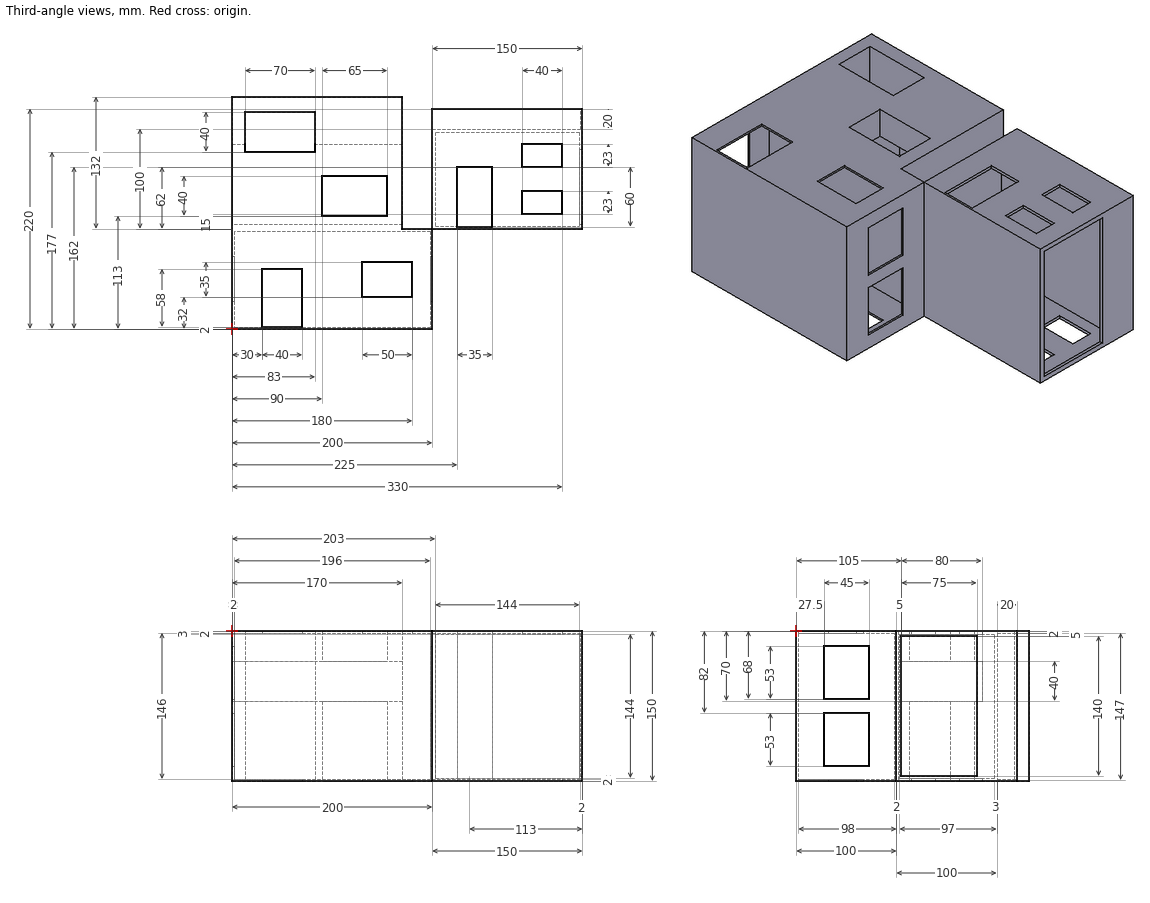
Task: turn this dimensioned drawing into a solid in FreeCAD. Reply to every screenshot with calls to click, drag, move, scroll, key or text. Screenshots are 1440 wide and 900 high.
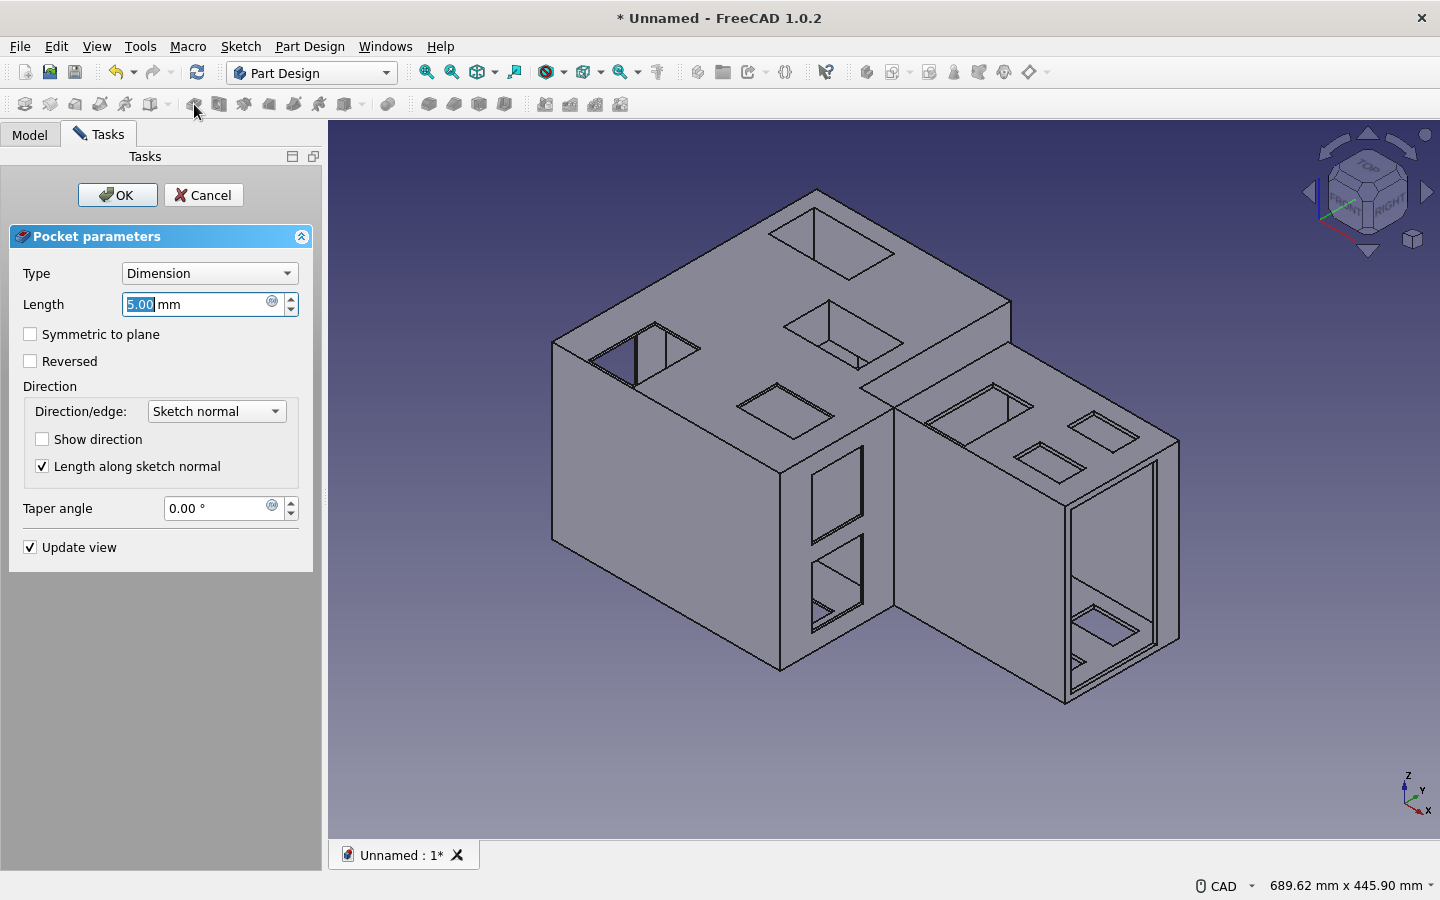
text(113)
key(Tab)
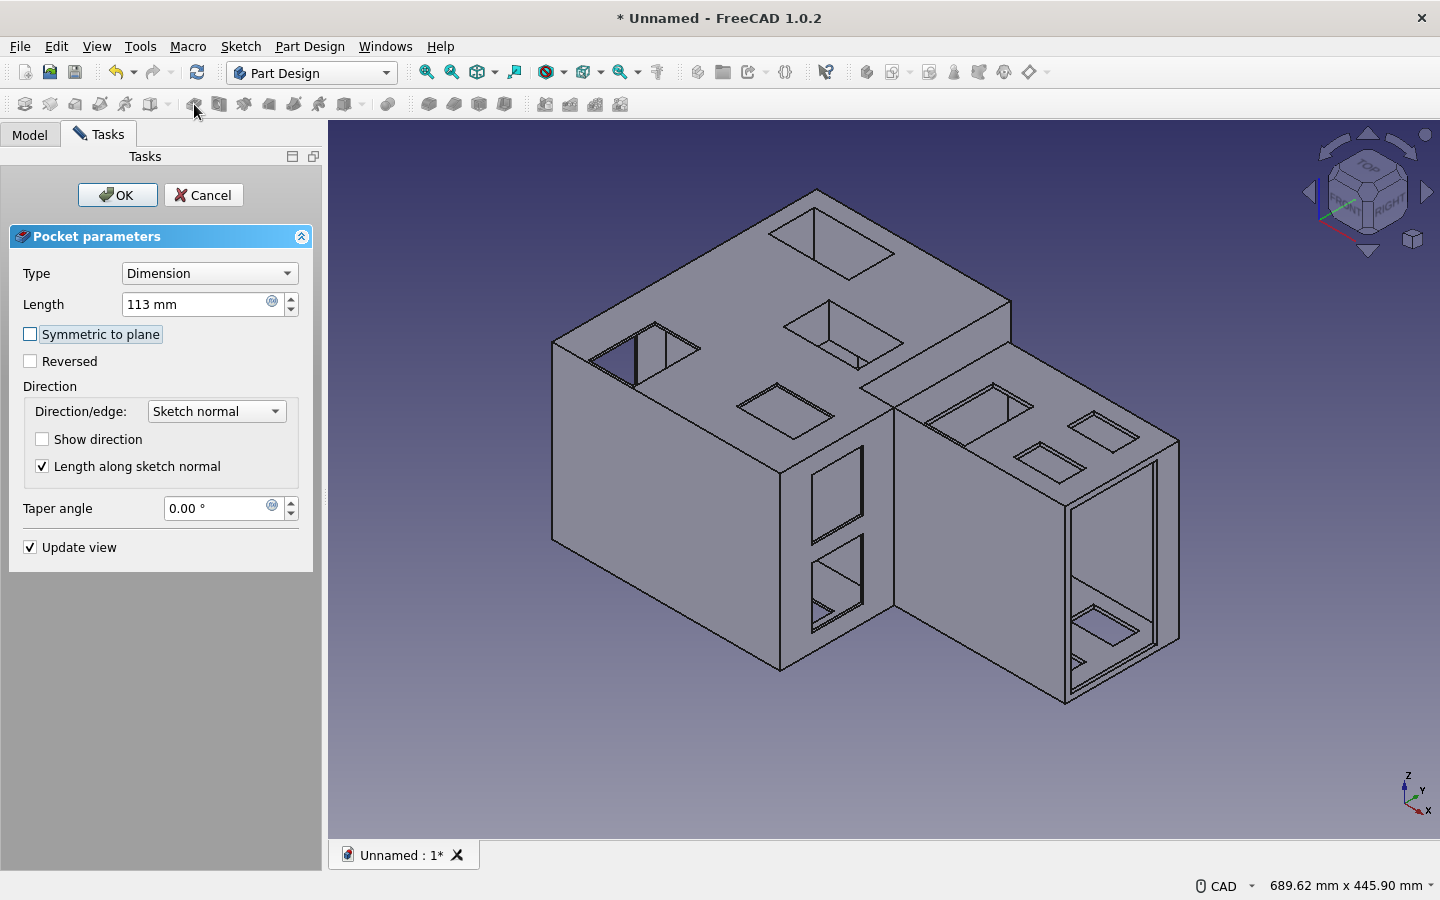
click(118, 195)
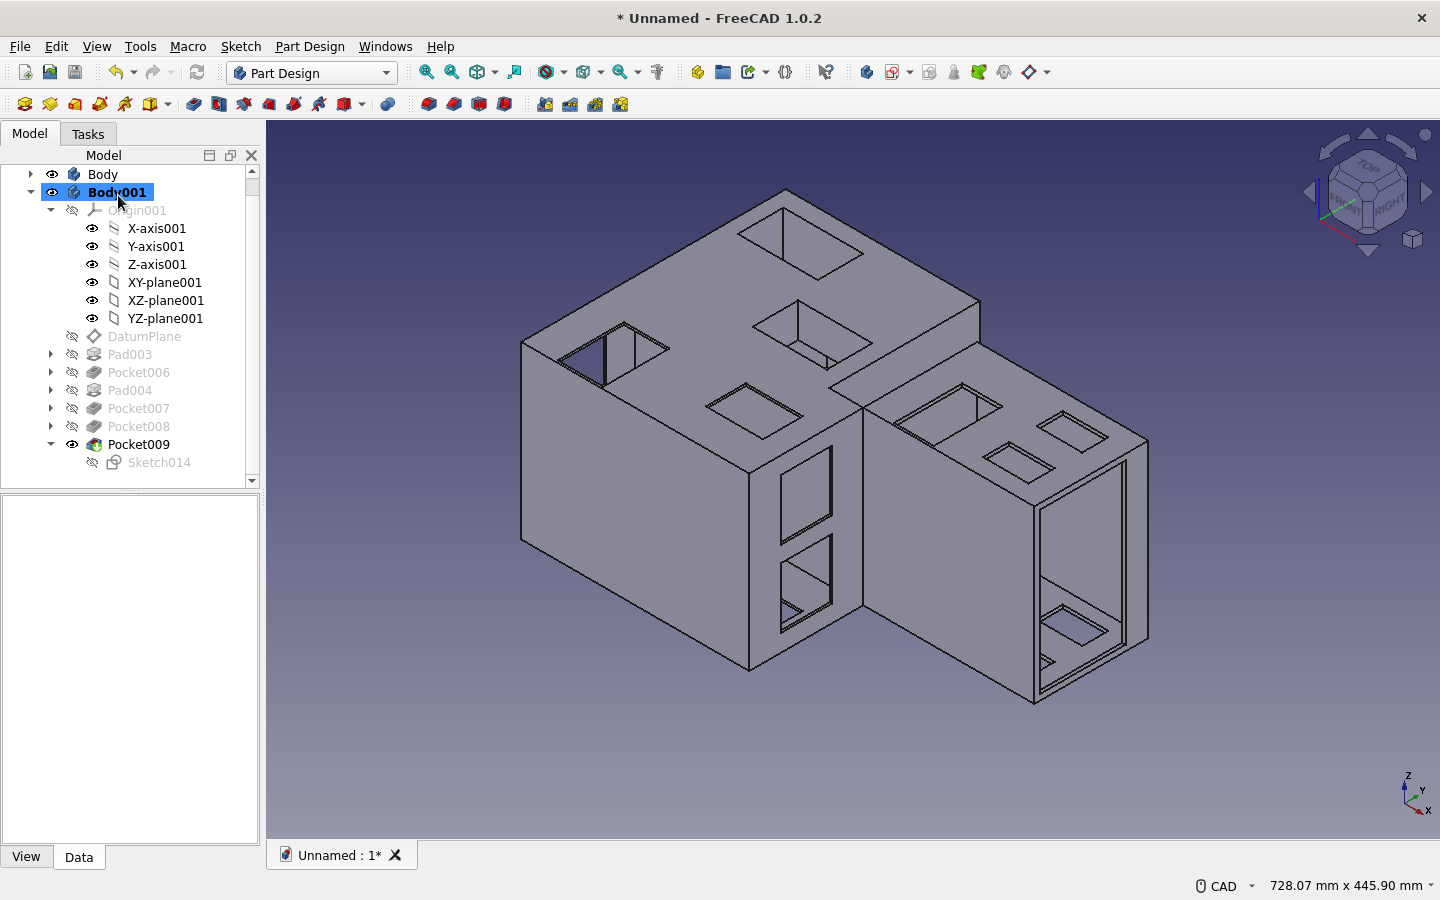
click(892, 72)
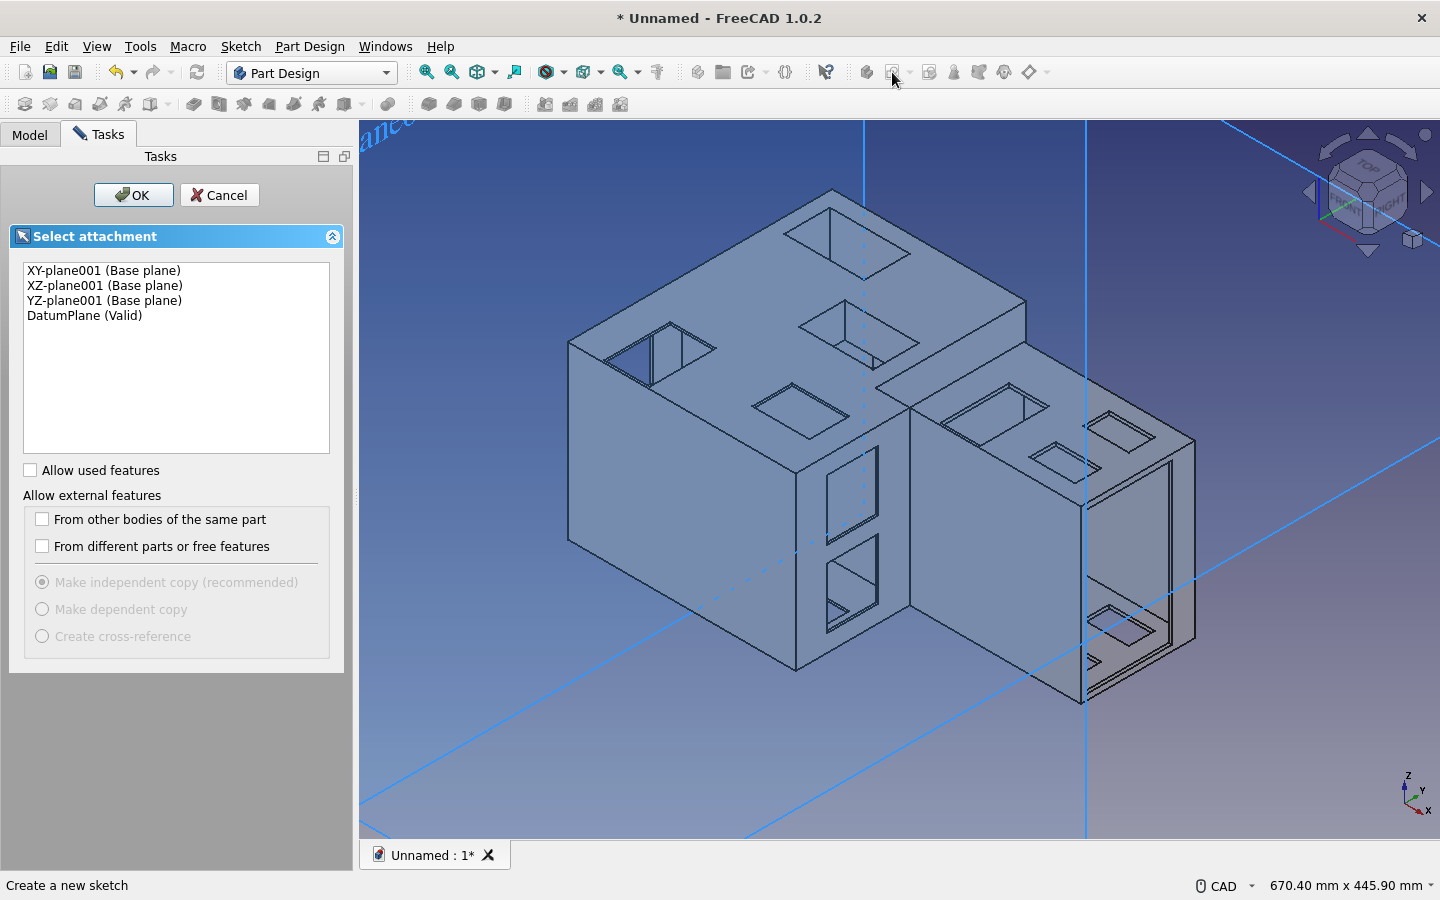
click(84, 270)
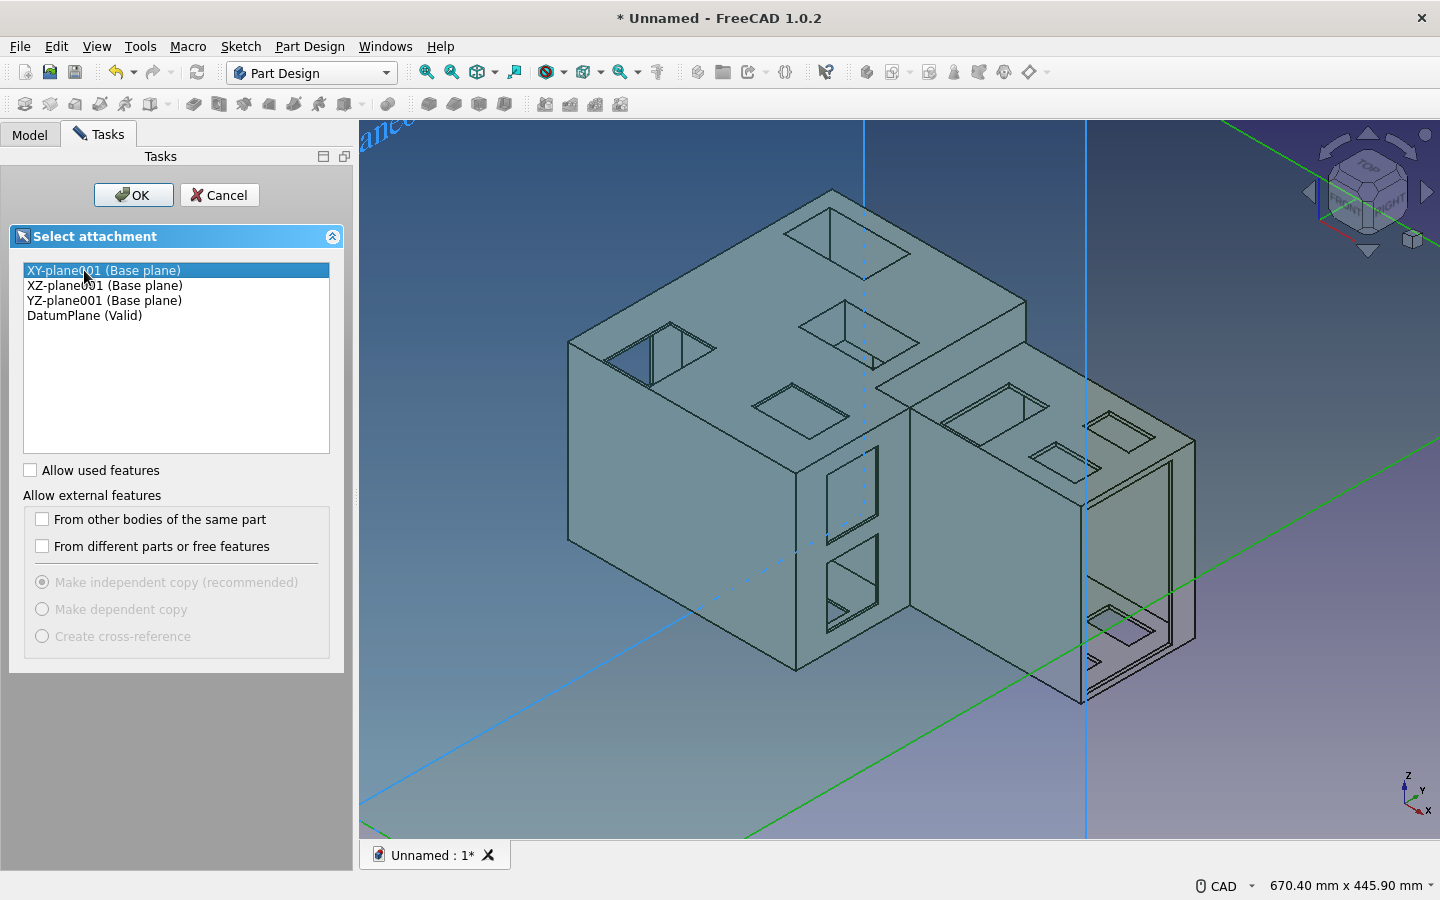
click(134, 195)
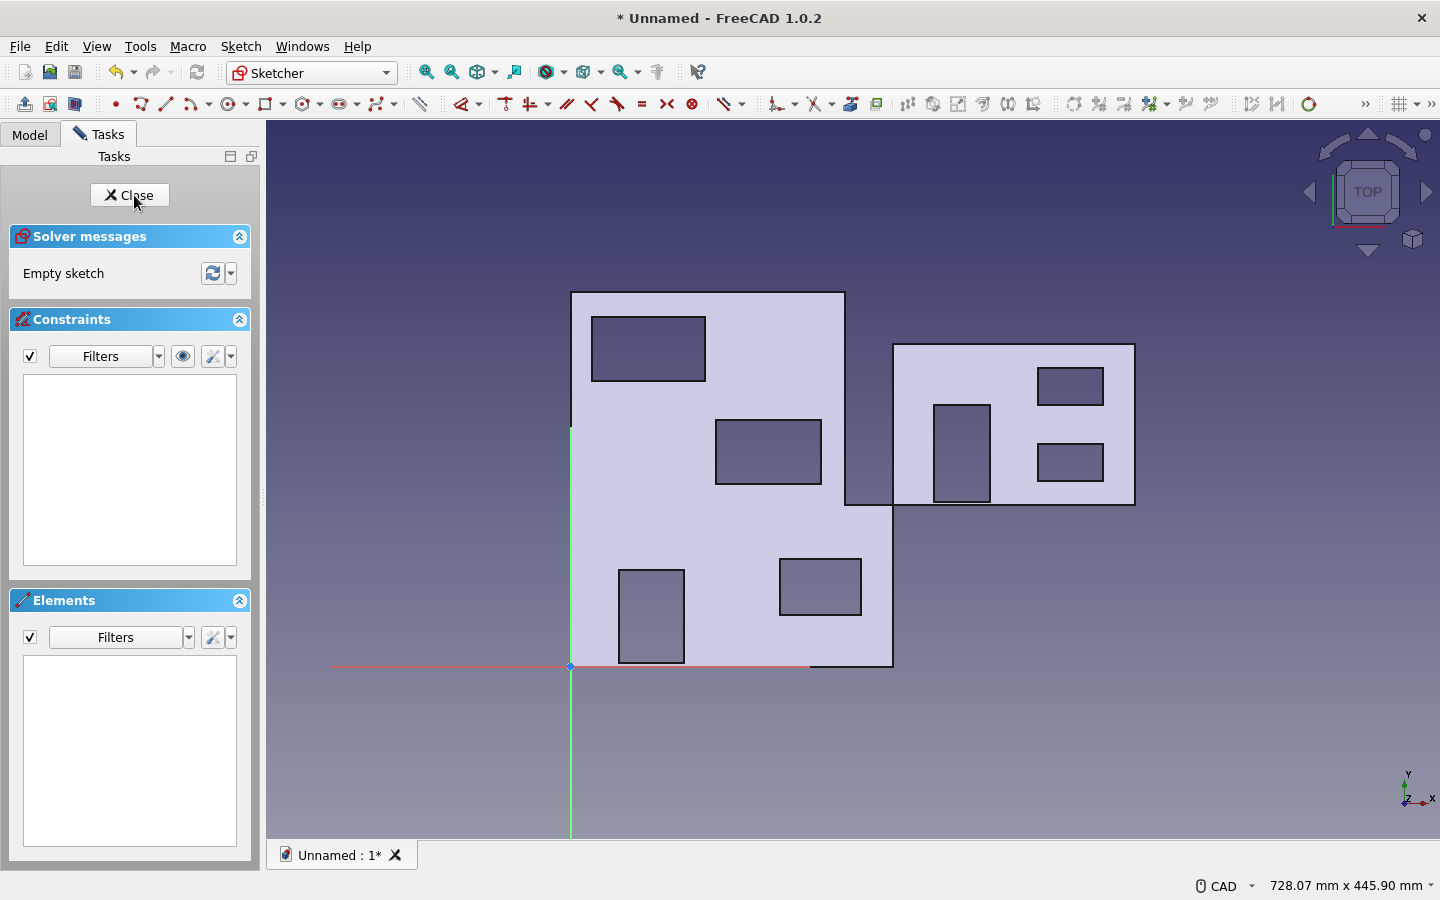
click(264, 104)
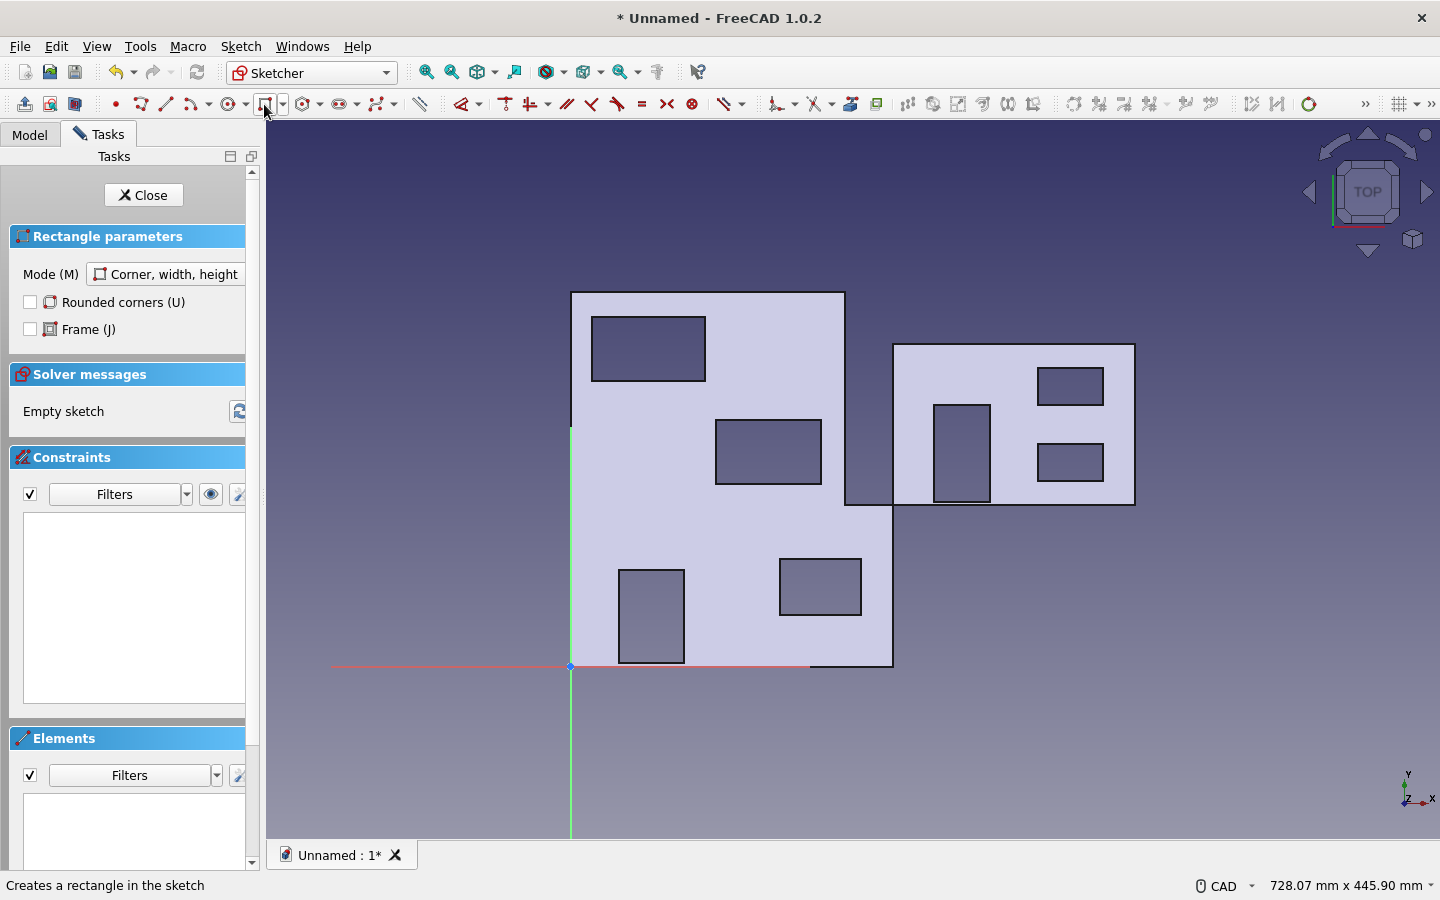
click(893, 312)
move(1135, 344)